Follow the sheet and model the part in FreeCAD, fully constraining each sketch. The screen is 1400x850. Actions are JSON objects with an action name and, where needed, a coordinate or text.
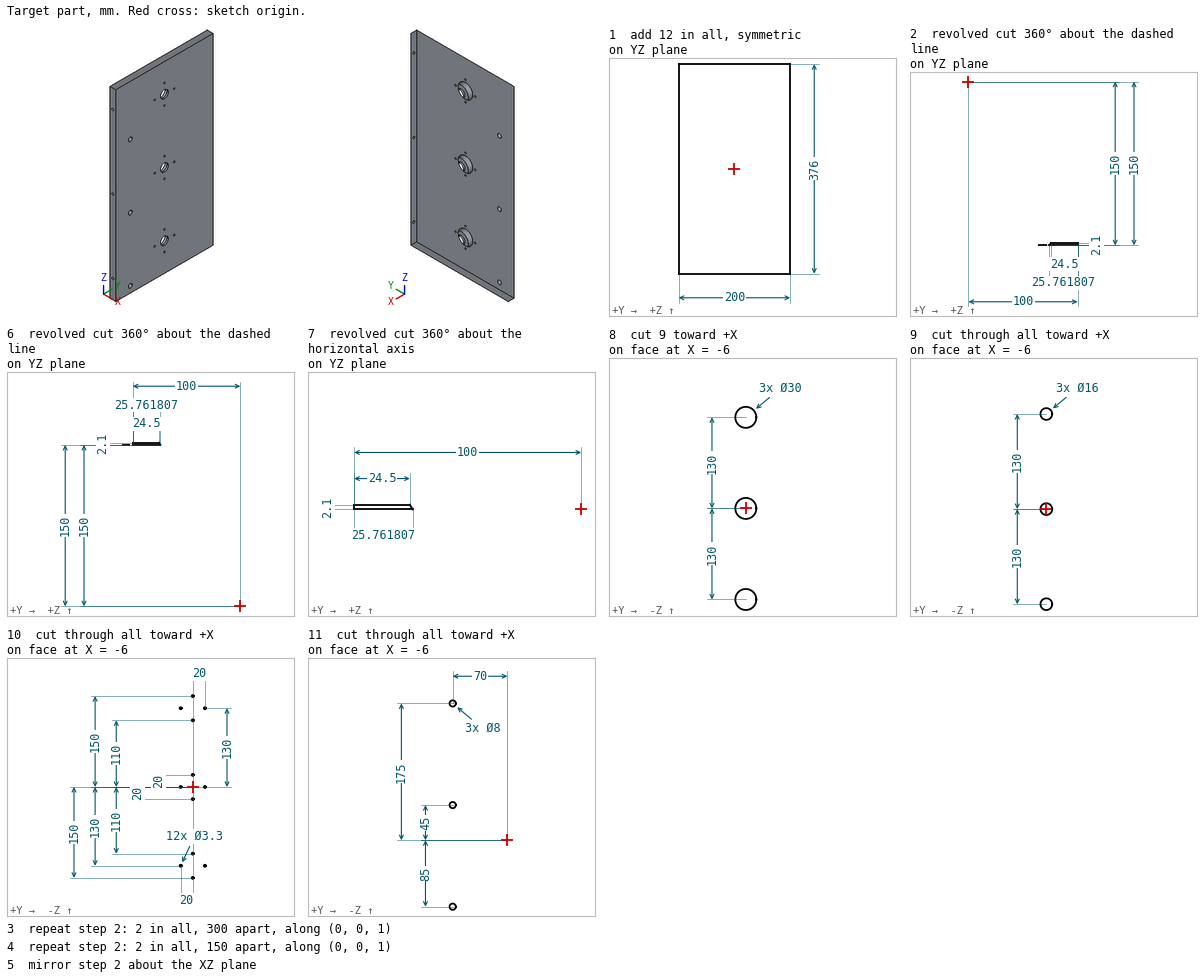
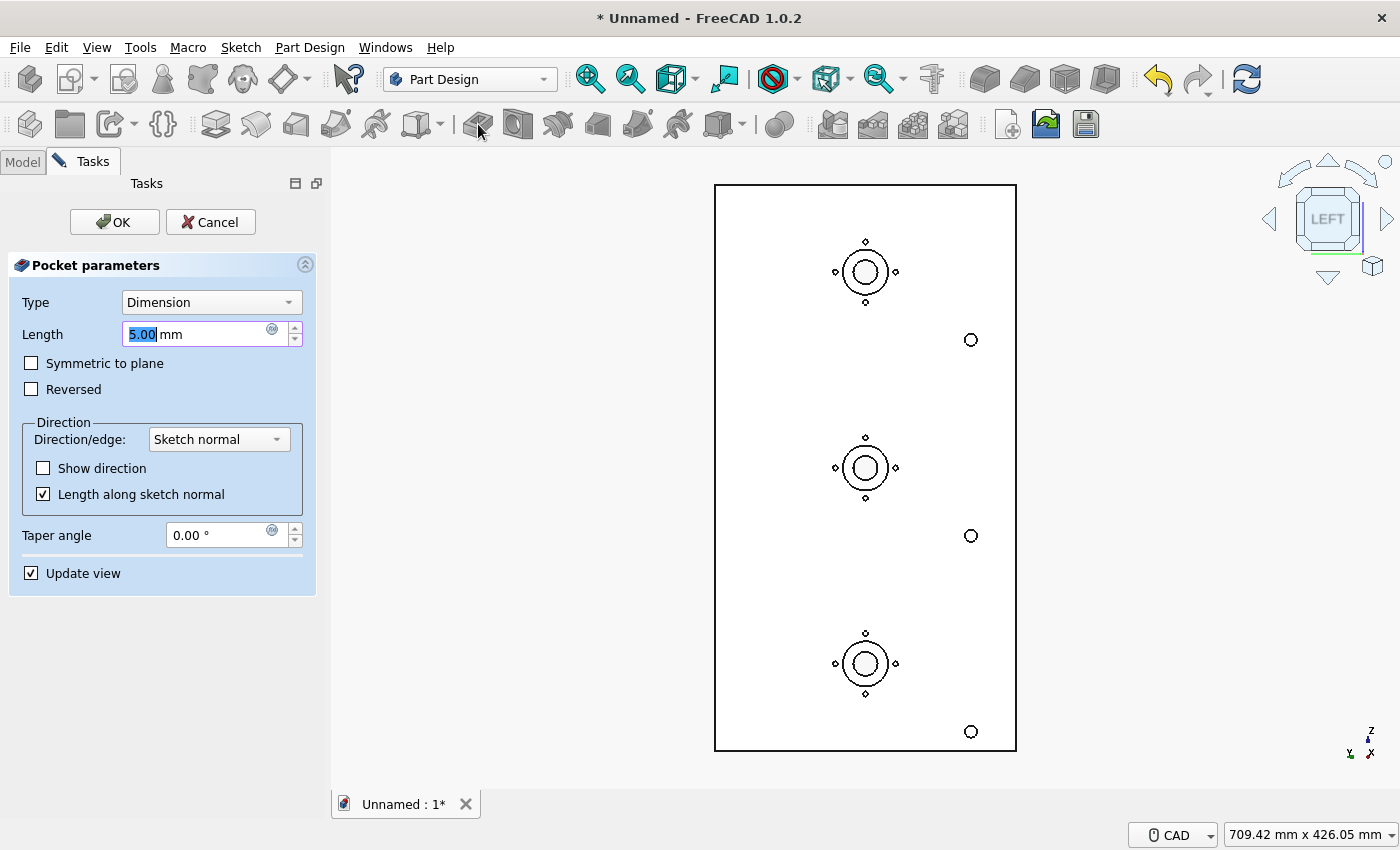
{"action": "left_click", "coordinate": [212, 302]}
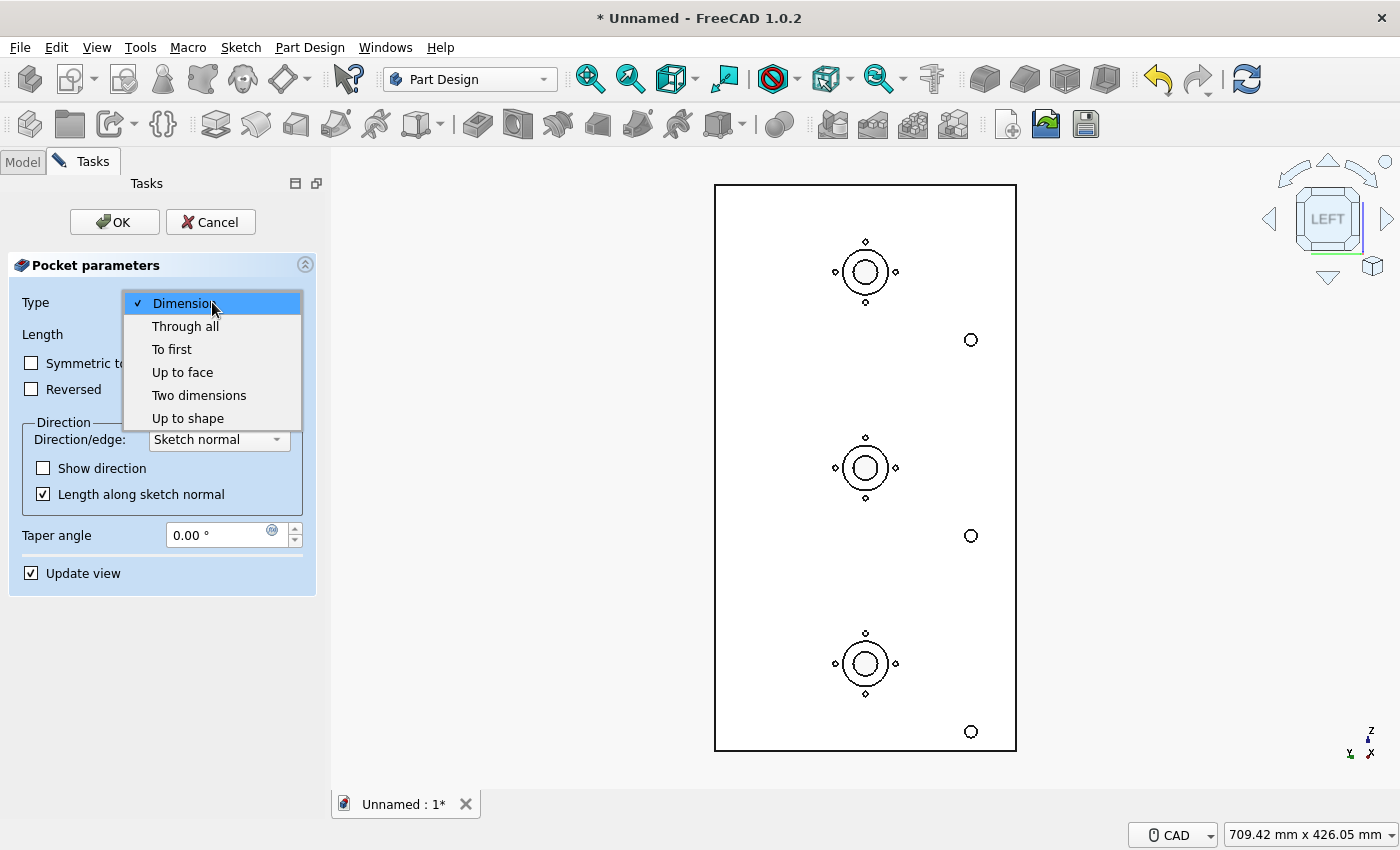
{"action": "left_click", "coordinate": [212, 326]}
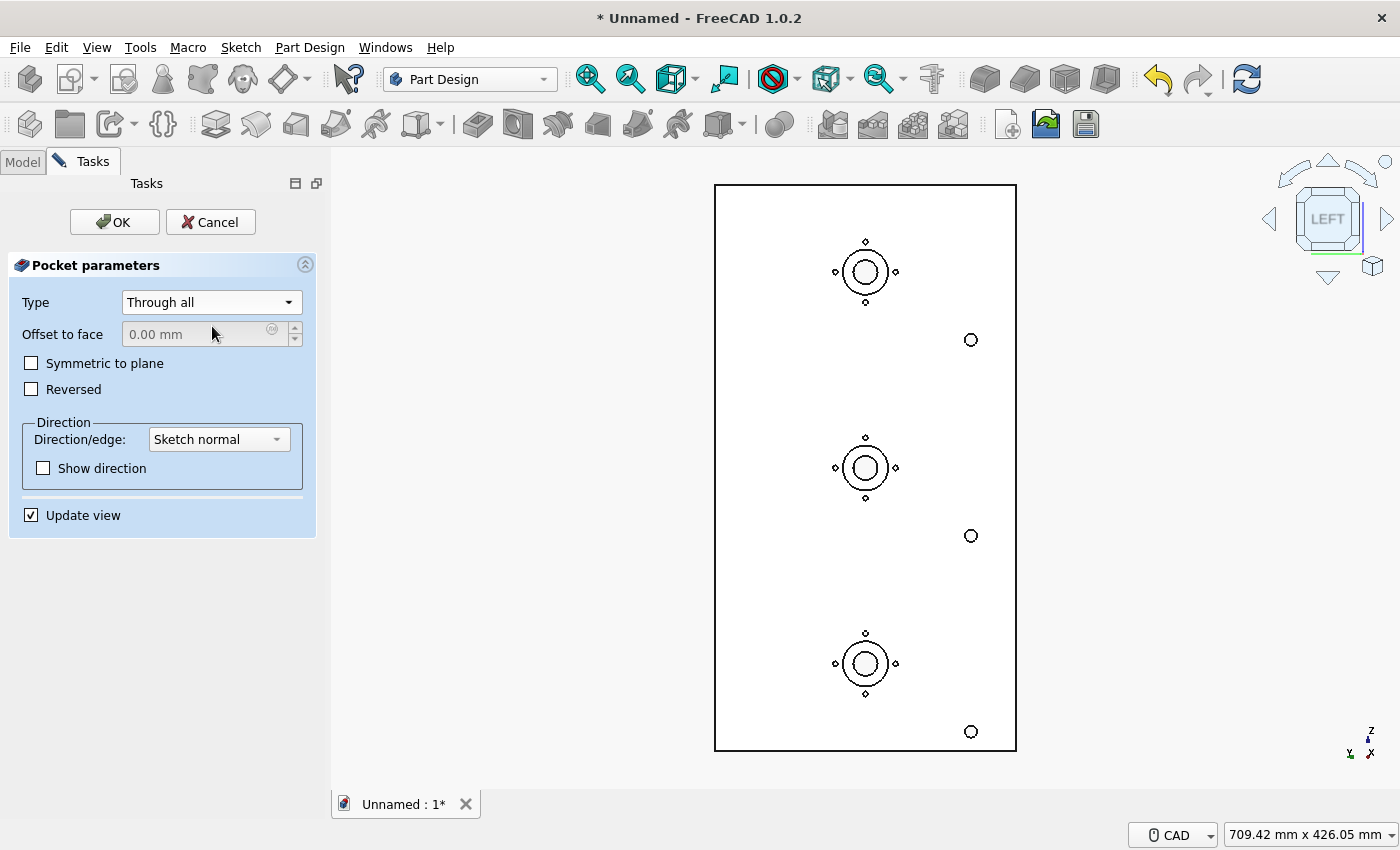
{"action": "left_click", "coordinate": [115, 222]}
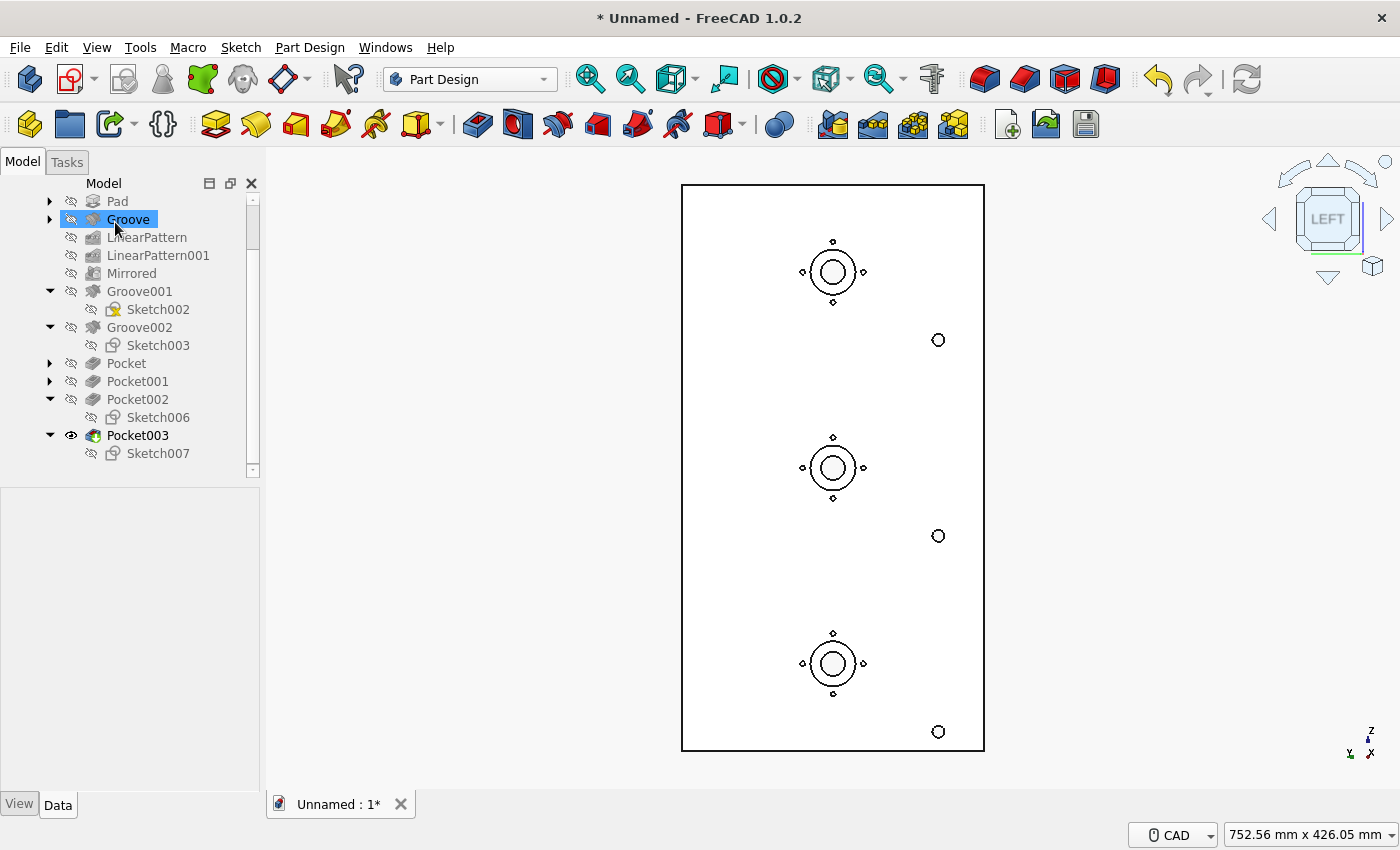
{"action": "key", "text": "0"}